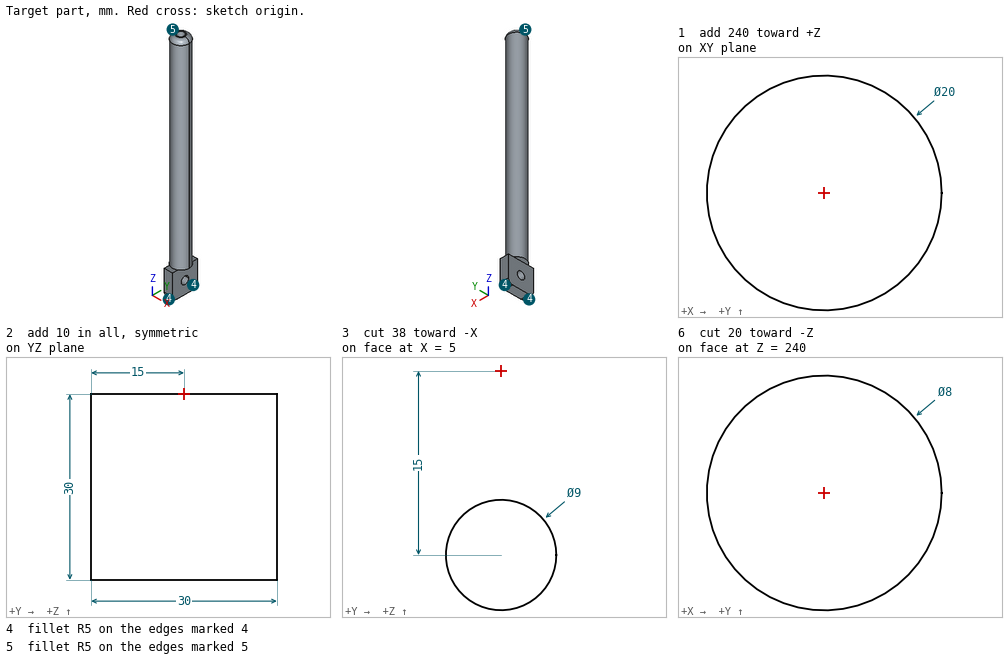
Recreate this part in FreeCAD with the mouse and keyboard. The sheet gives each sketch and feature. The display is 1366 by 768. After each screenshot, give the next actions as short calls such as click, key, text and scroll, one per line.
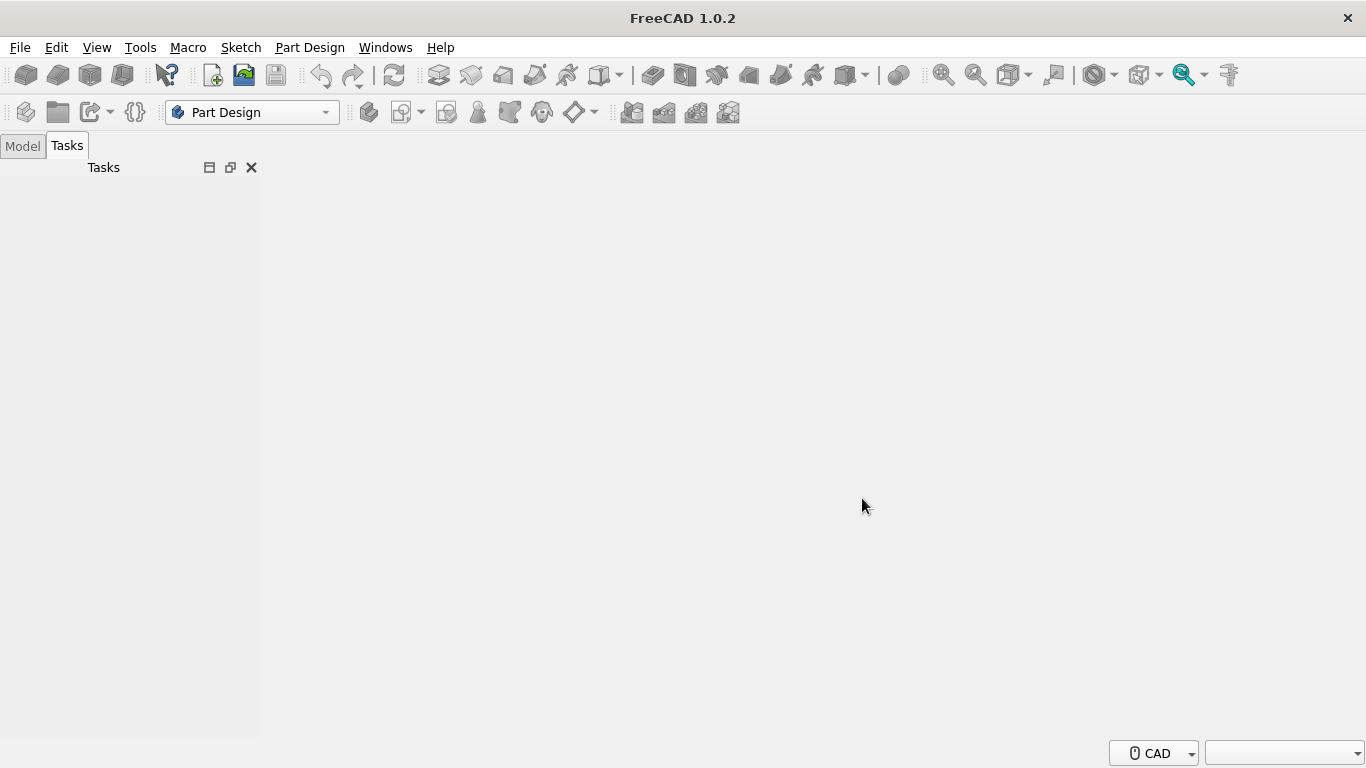
key(ctrl+n)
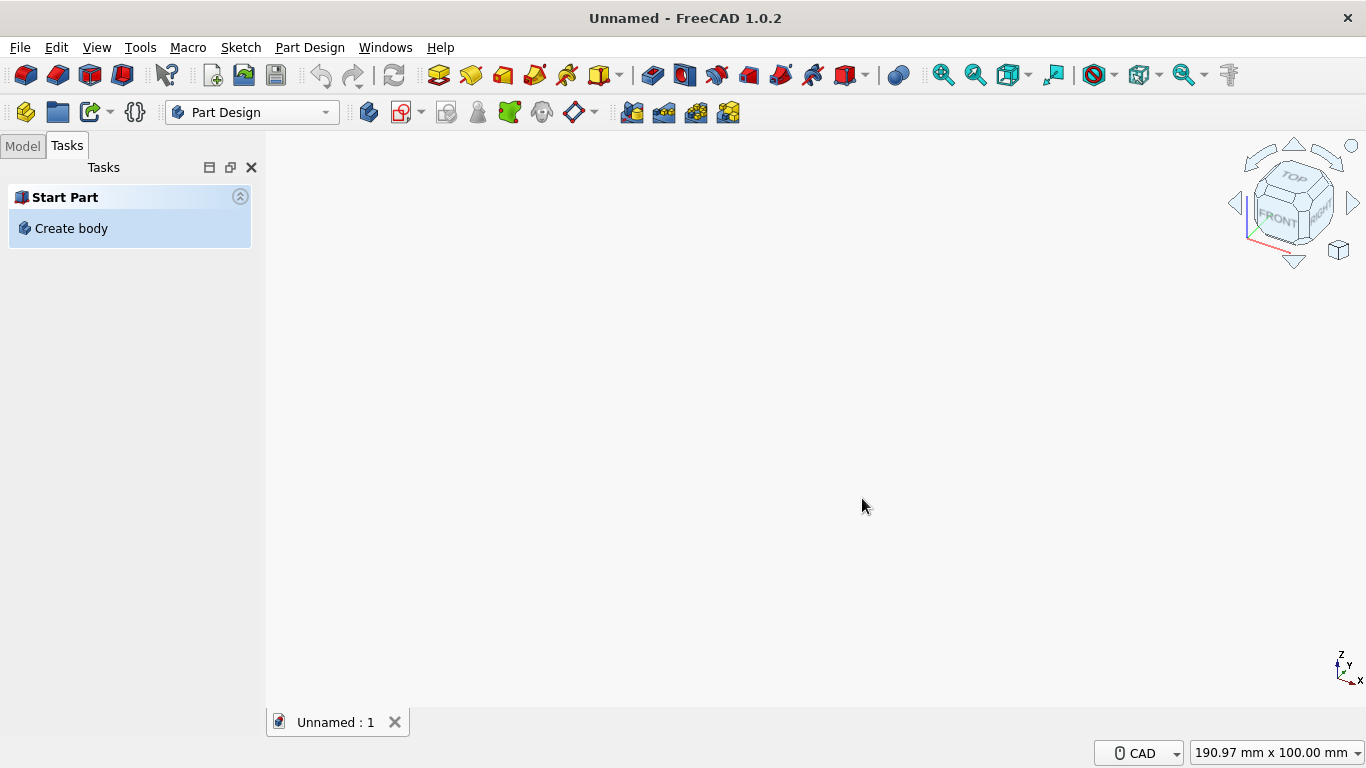
click(402, 112)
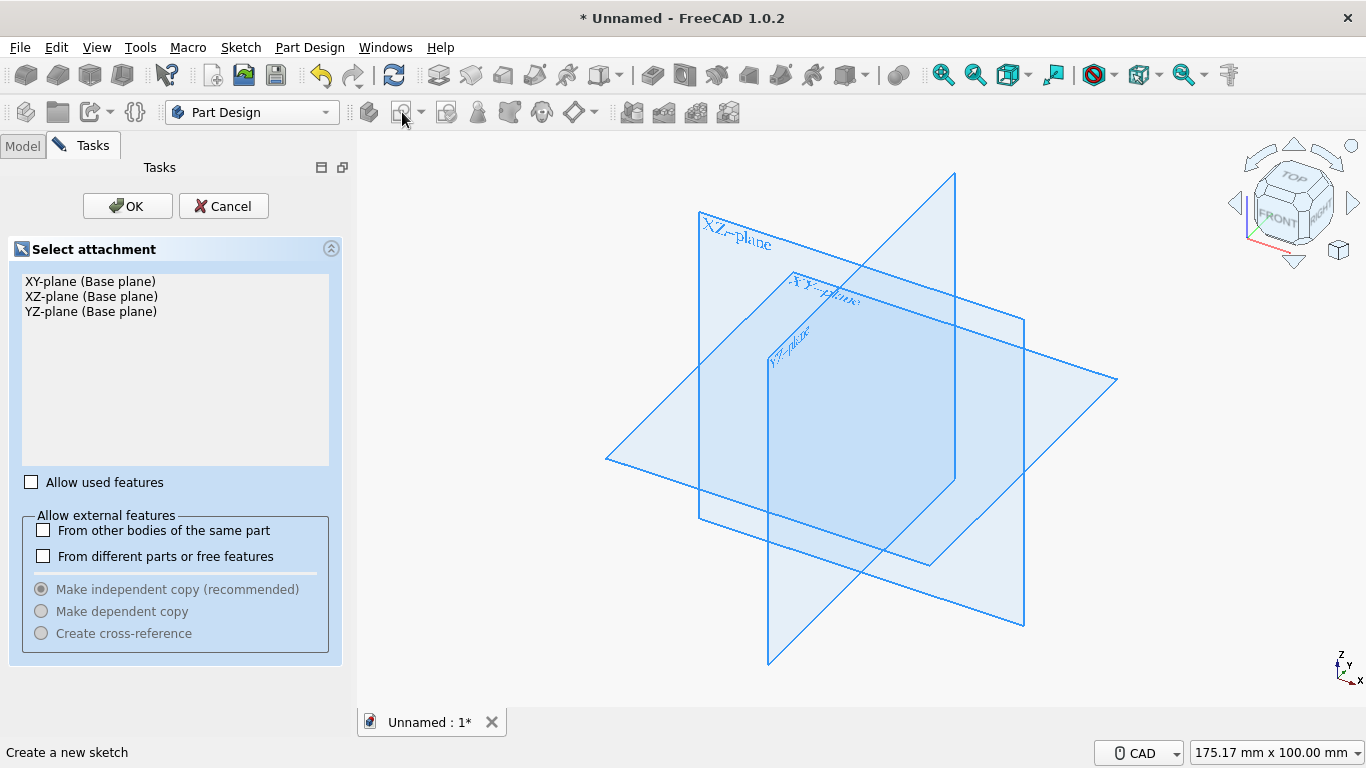
click(82, 282)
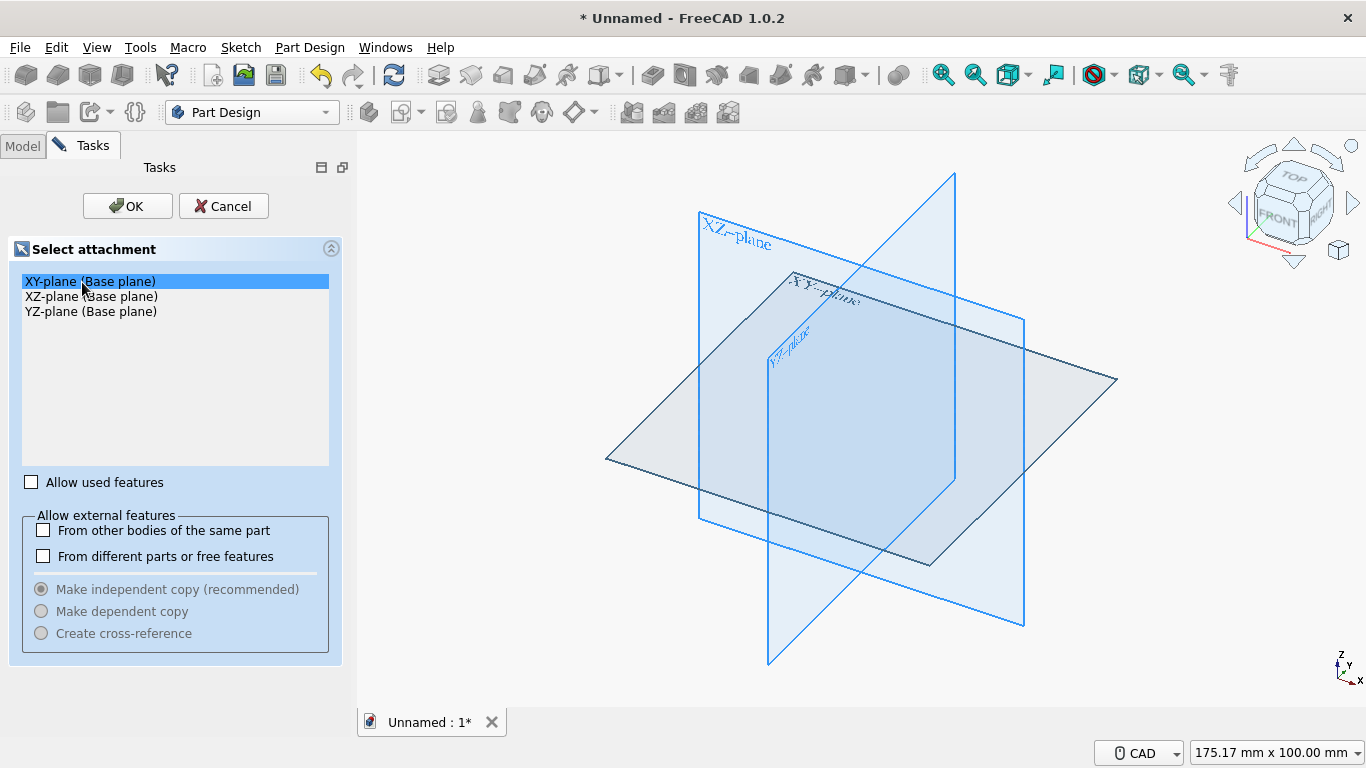
click(128, 206)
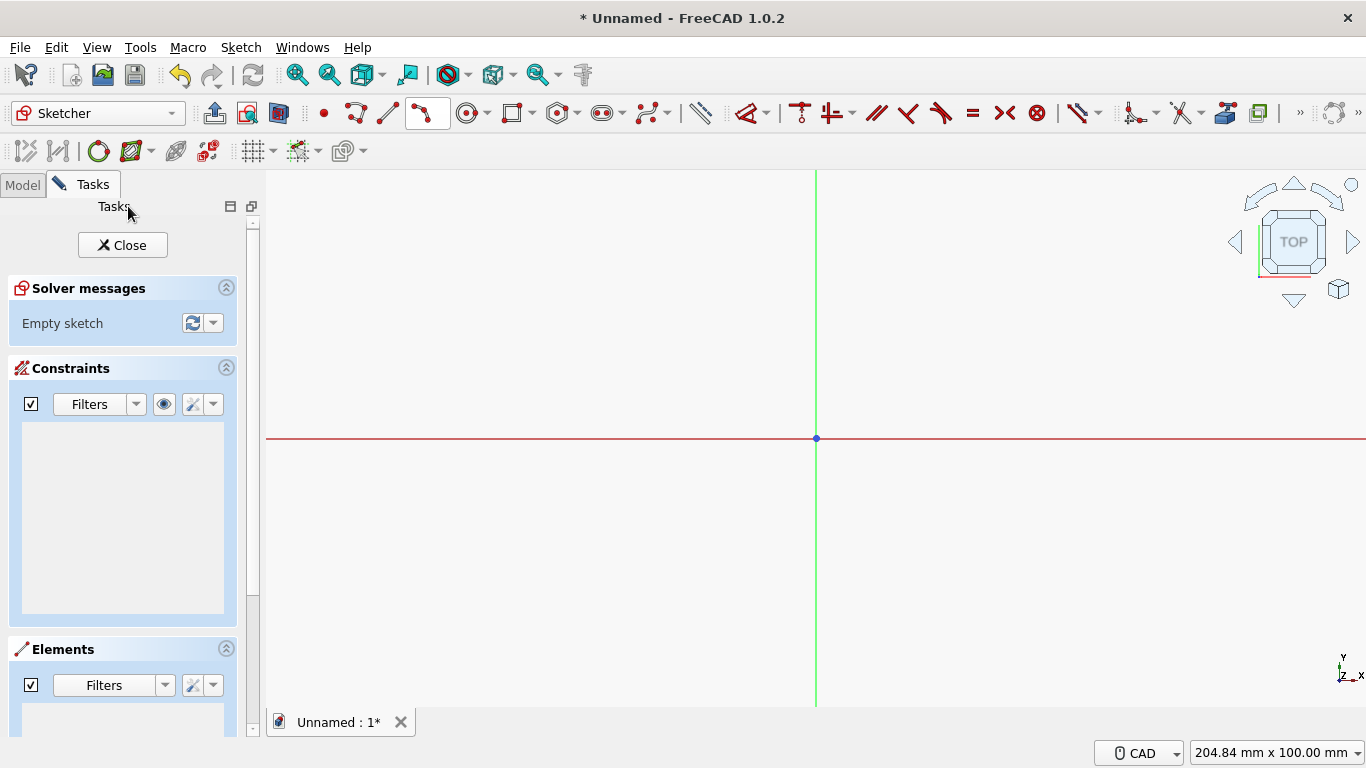
scroll(846, 438, up, 6)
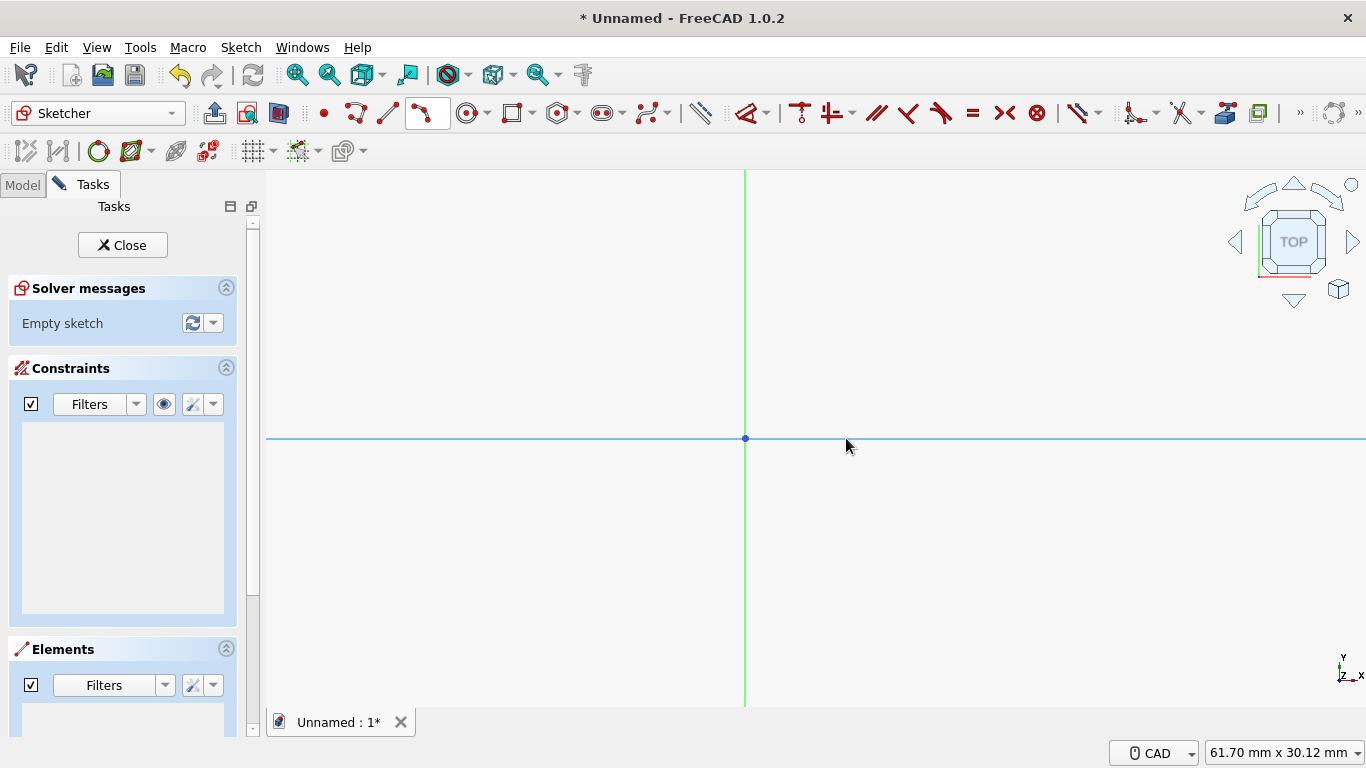
key(g)
key(c)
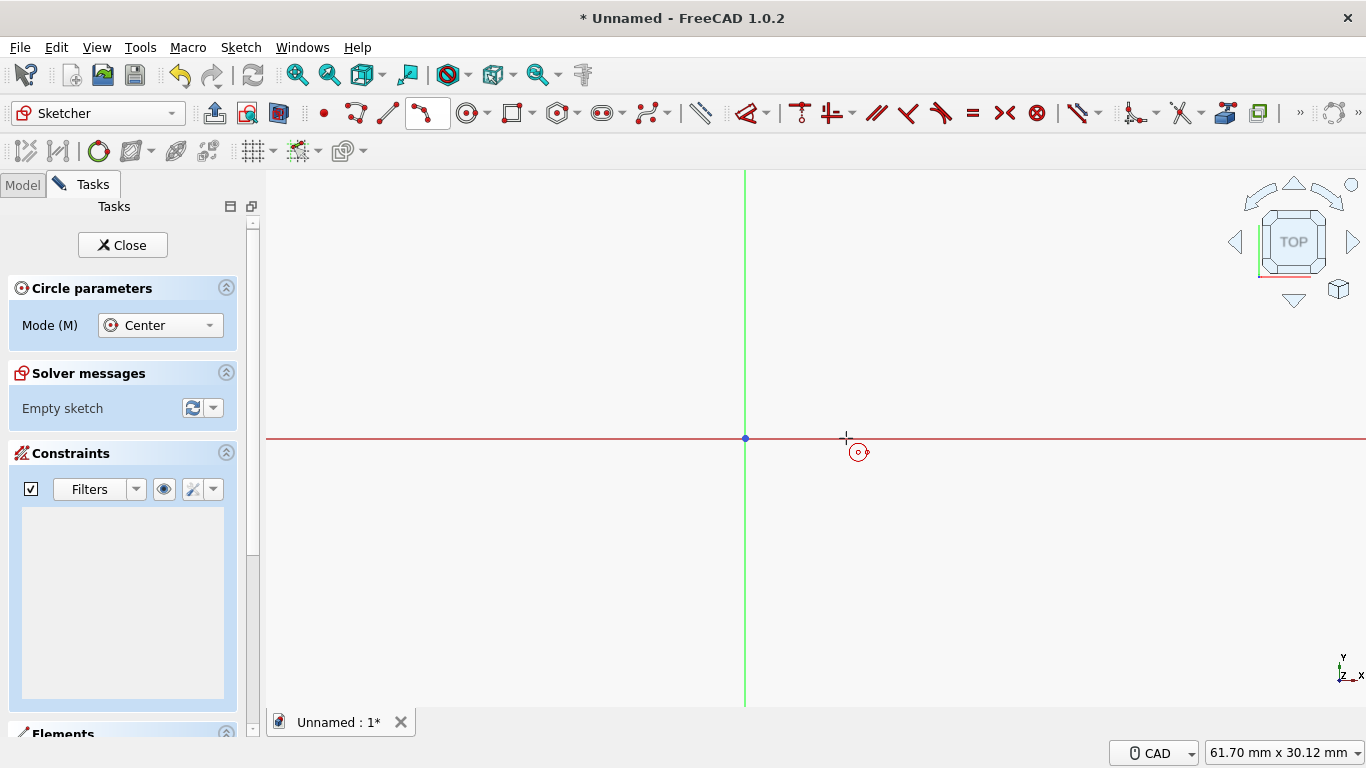
click(745, 438)
click(871, 312)
key(Escape)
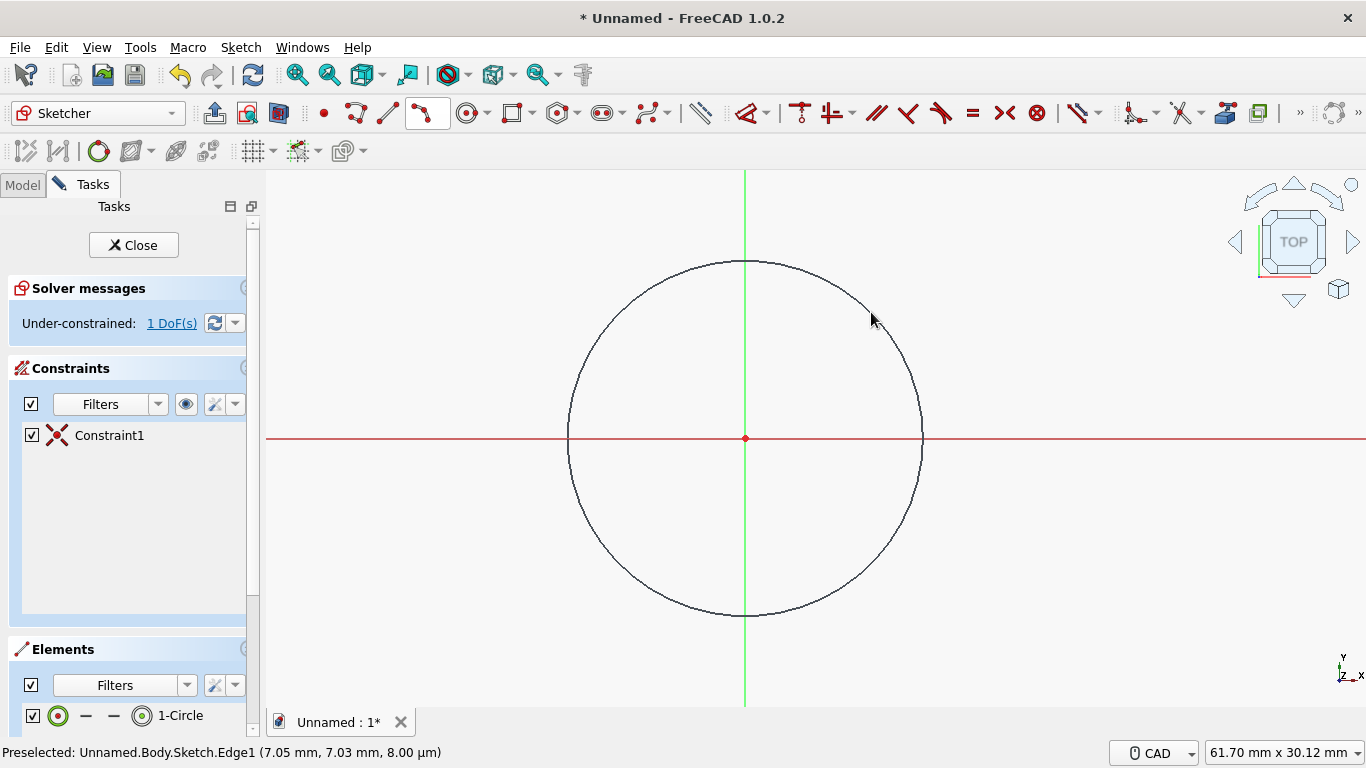
key(d)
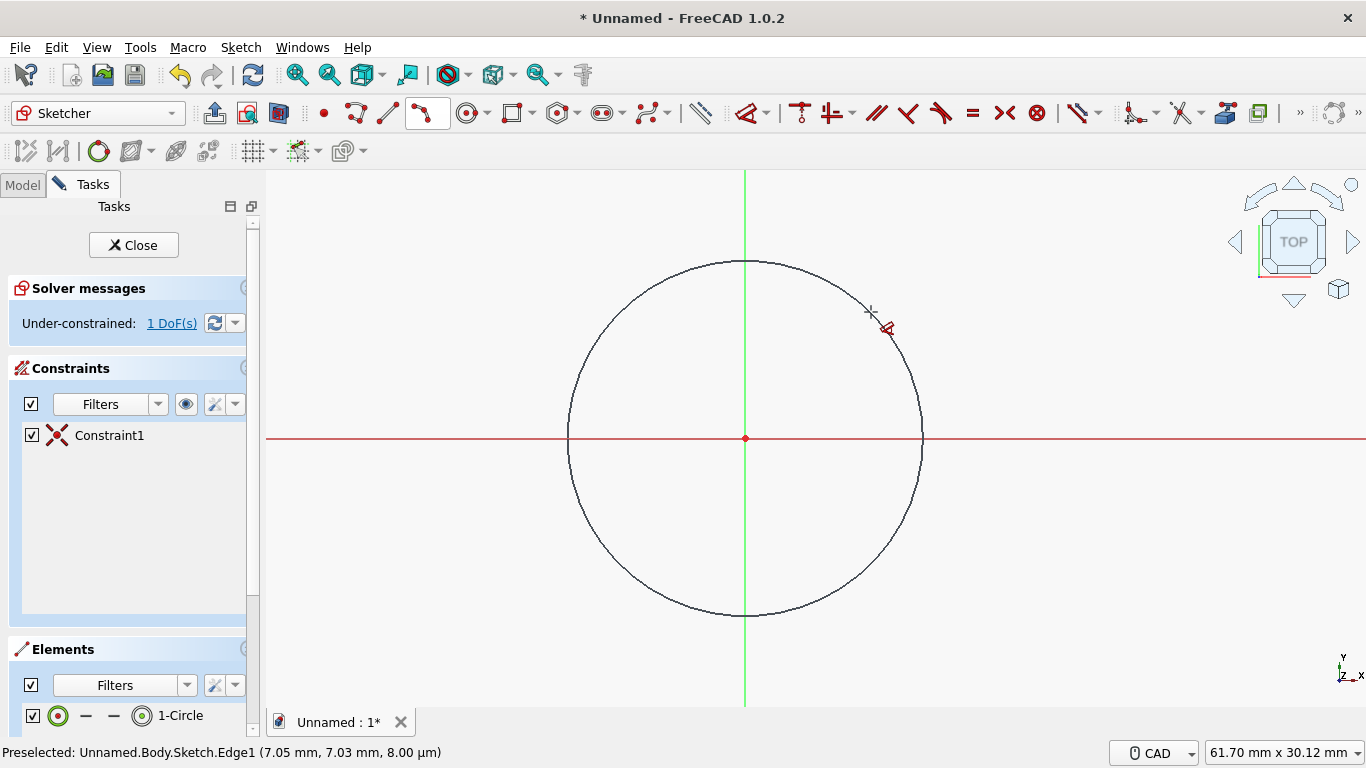
click(870, 312)
click(892, 289)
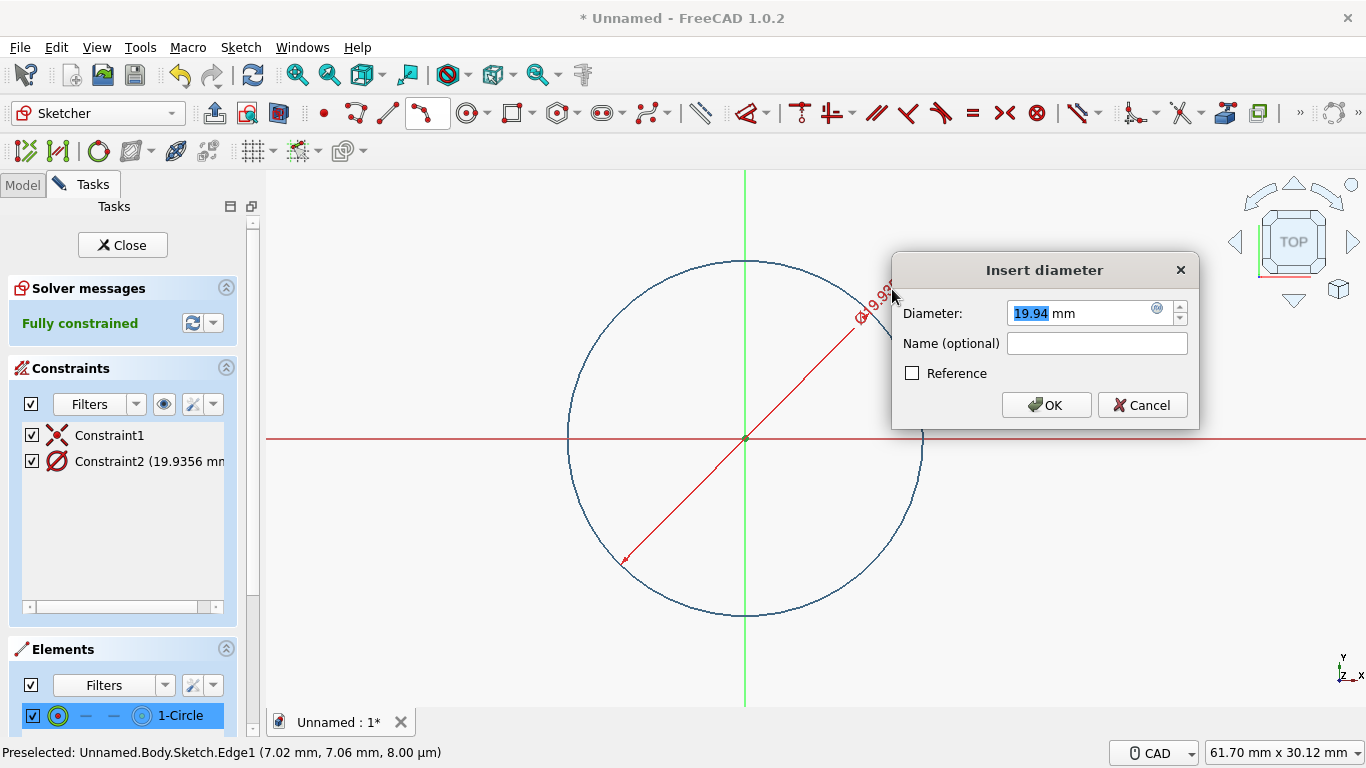
text(20)
key(Return)
key(Escape)